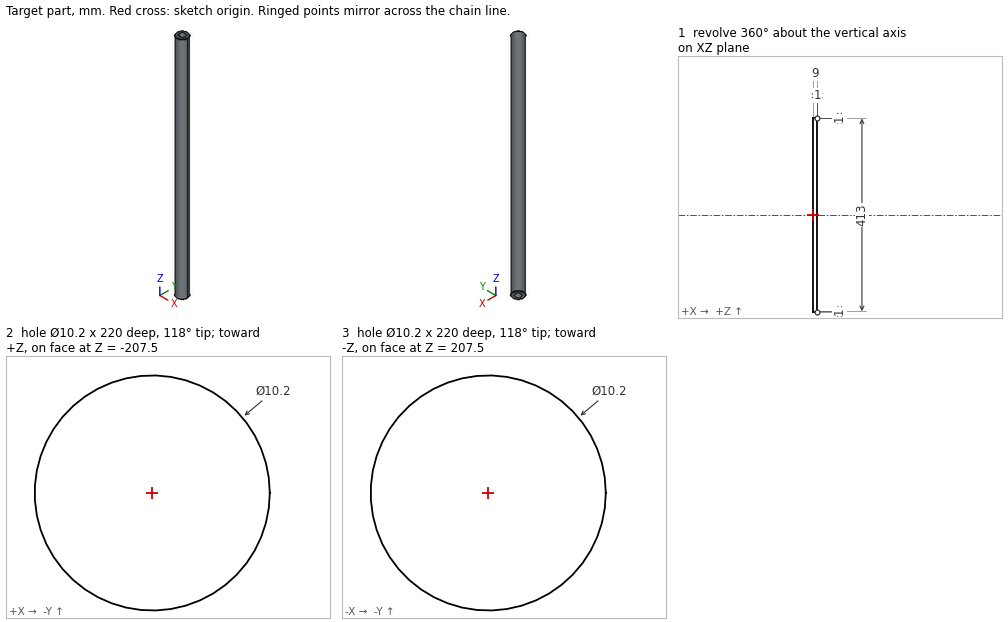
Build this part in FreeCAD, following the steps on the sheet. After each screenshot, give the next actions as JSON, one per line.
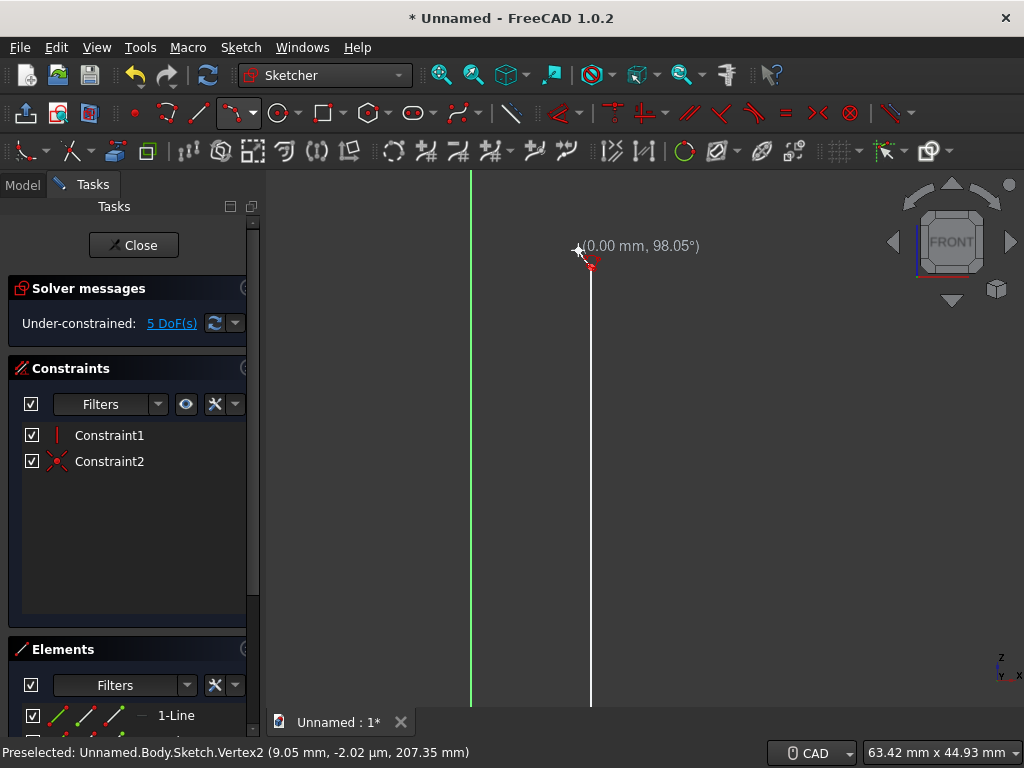
{"action": "scroll", "coordinate": [580, 255], "scroll_direction": "down", "scroll_amount": 13}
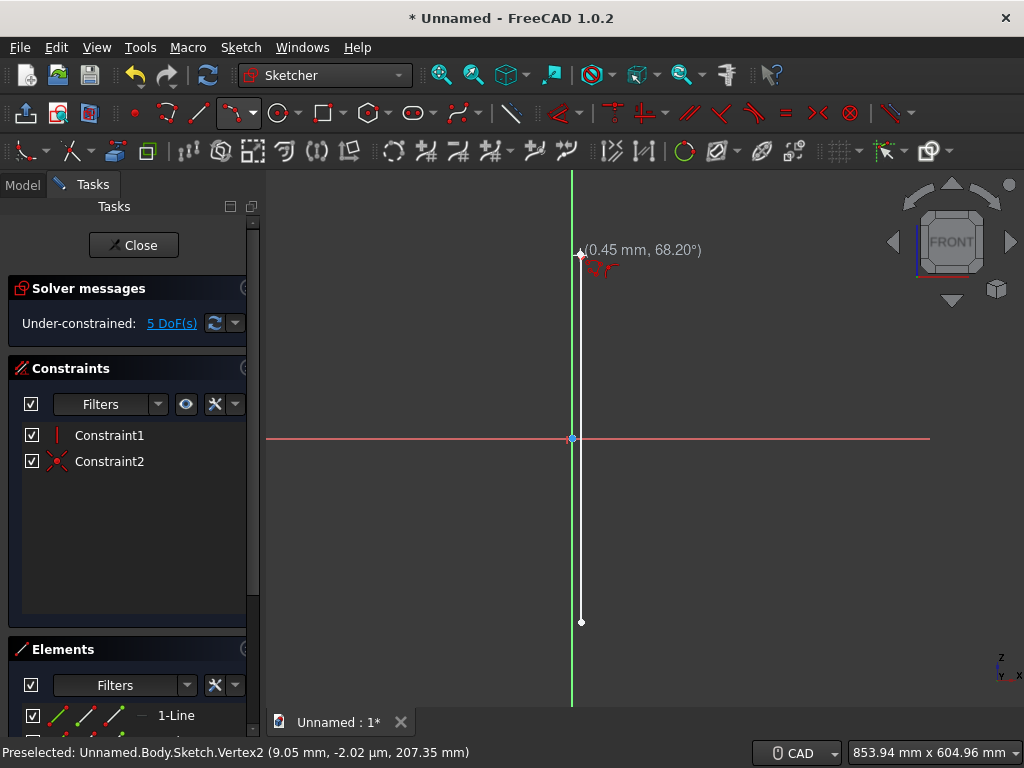
{"action": "scroll", "coordinate": [572, 255], "scroll_direction": "up", "scroll_amount": 4}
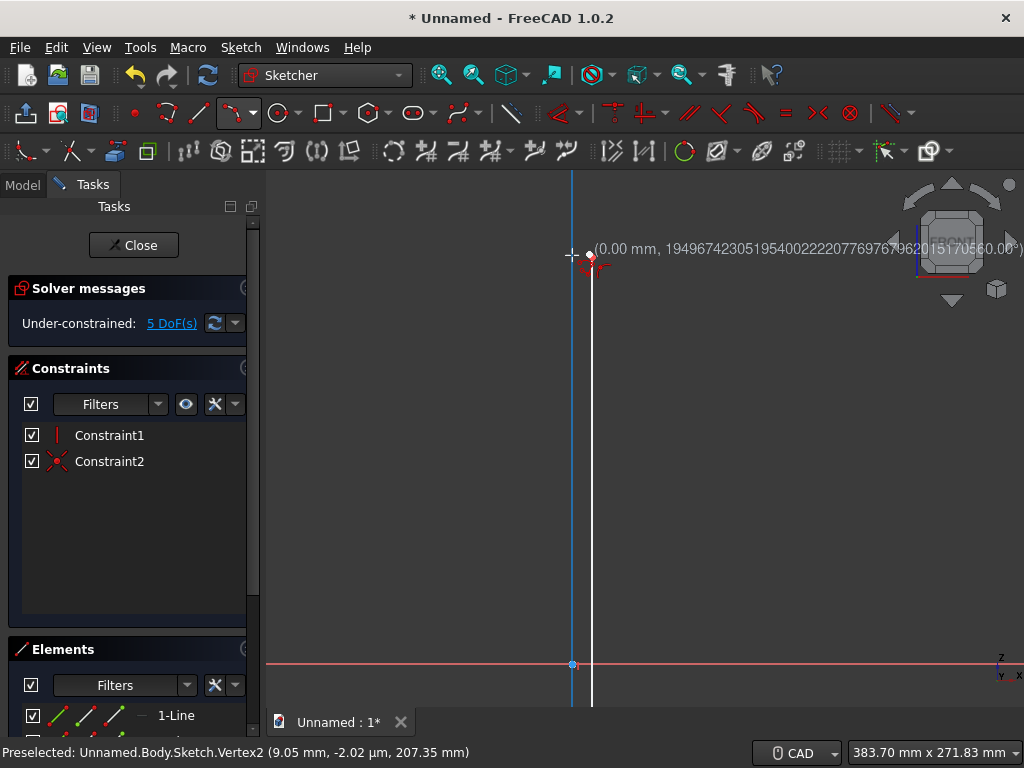
{"action": "left_click", "coordinate": [572, 254]}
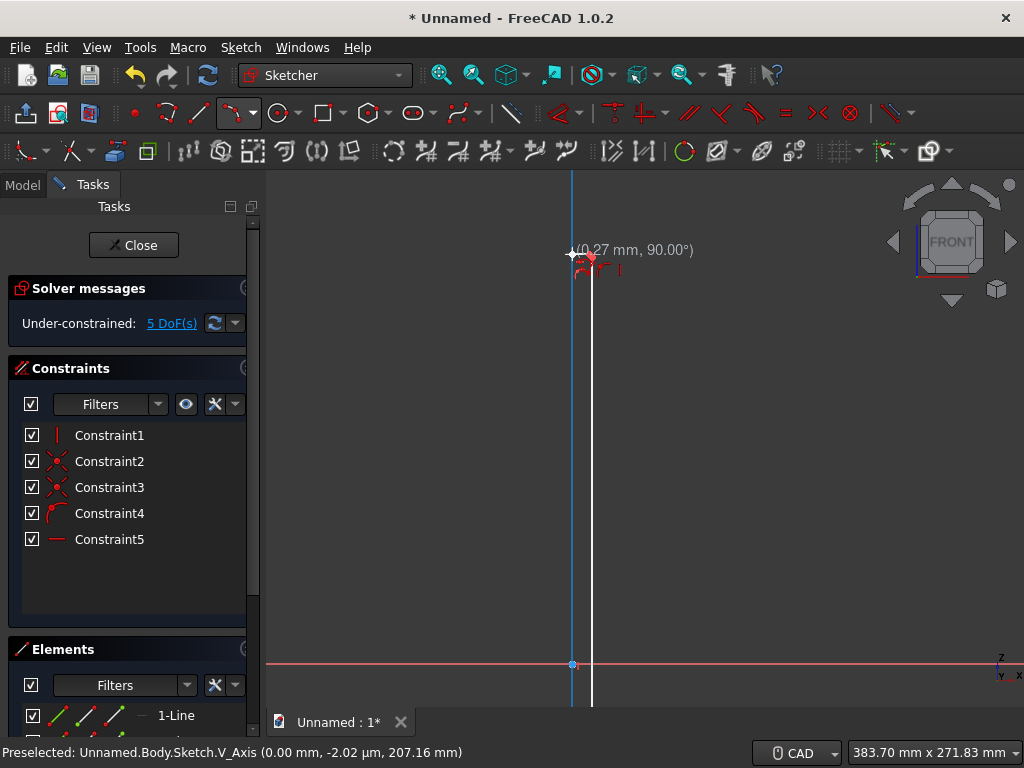
{"action": "scroll", "coordinate": [572, 254], "scroll_direction": "down", "scroll_amount": 4}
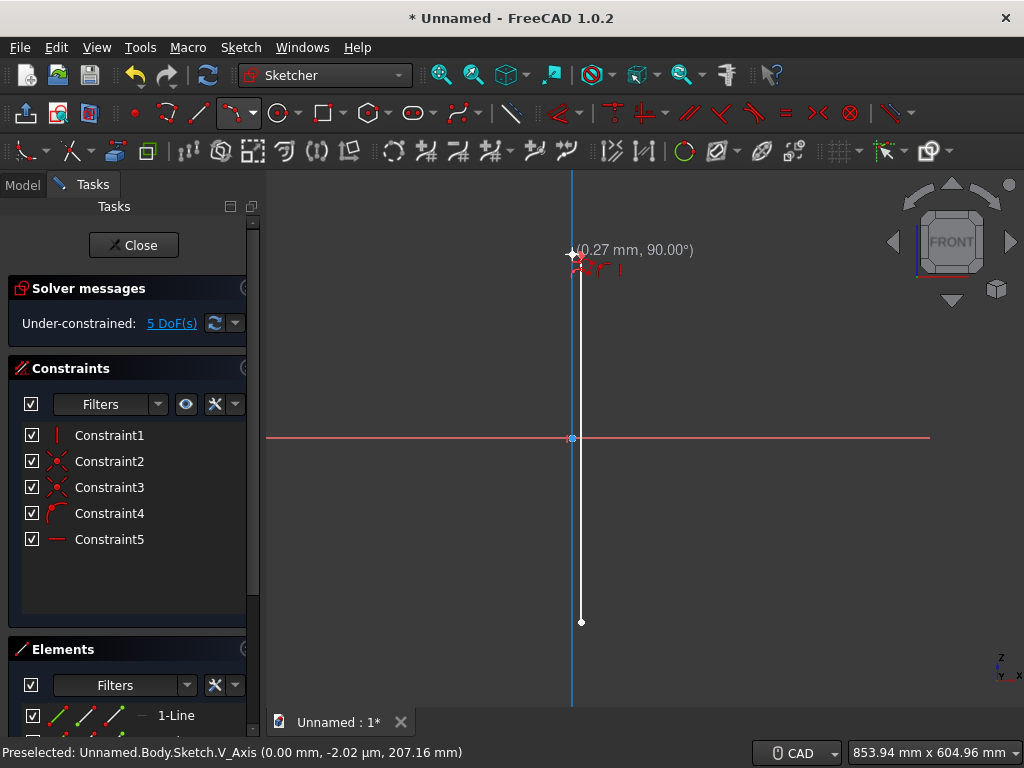
{"action": "scroll", "coordinate": [572, 623], "scroll_direction": "up", "scroll_amount": 3}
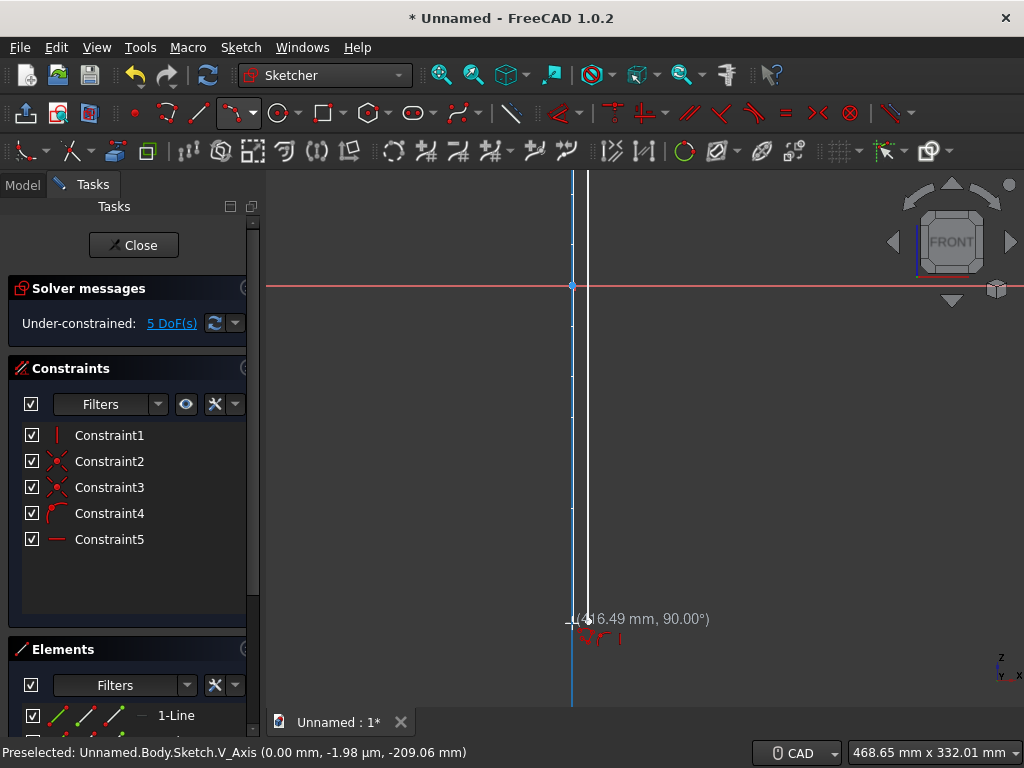
{"action": "left_click", "coordinate": [581, 622]}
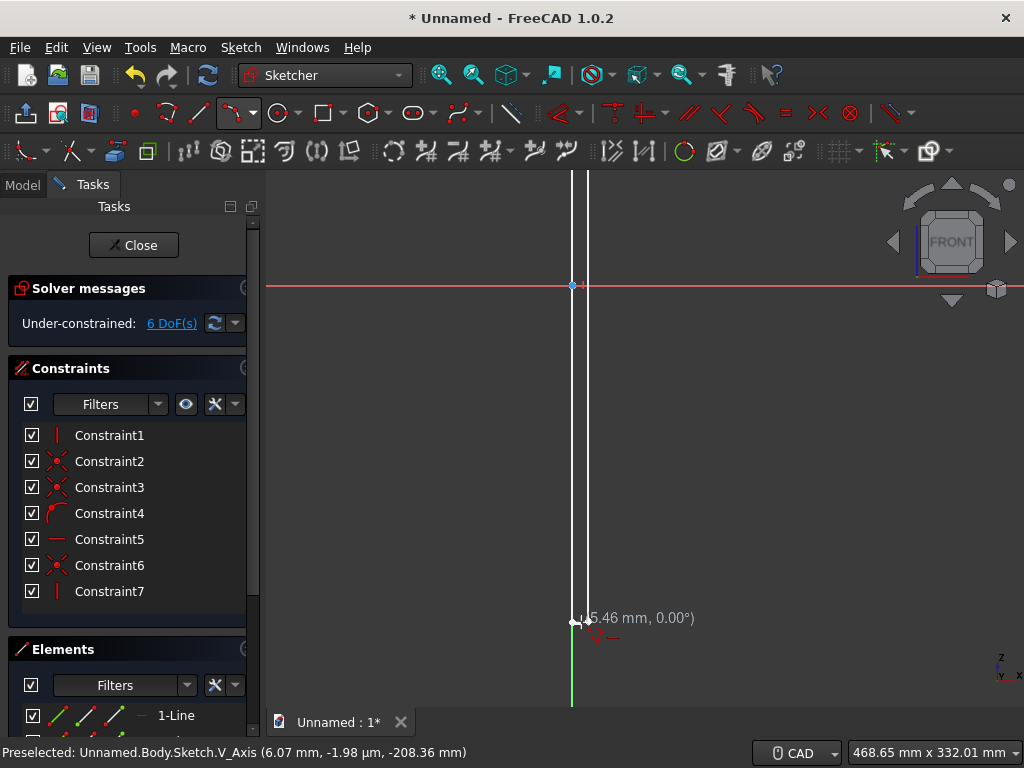
{"action": "scroll", "coordinate": [587, 622], "scroll_direction": "up", "scroll_amount": 10}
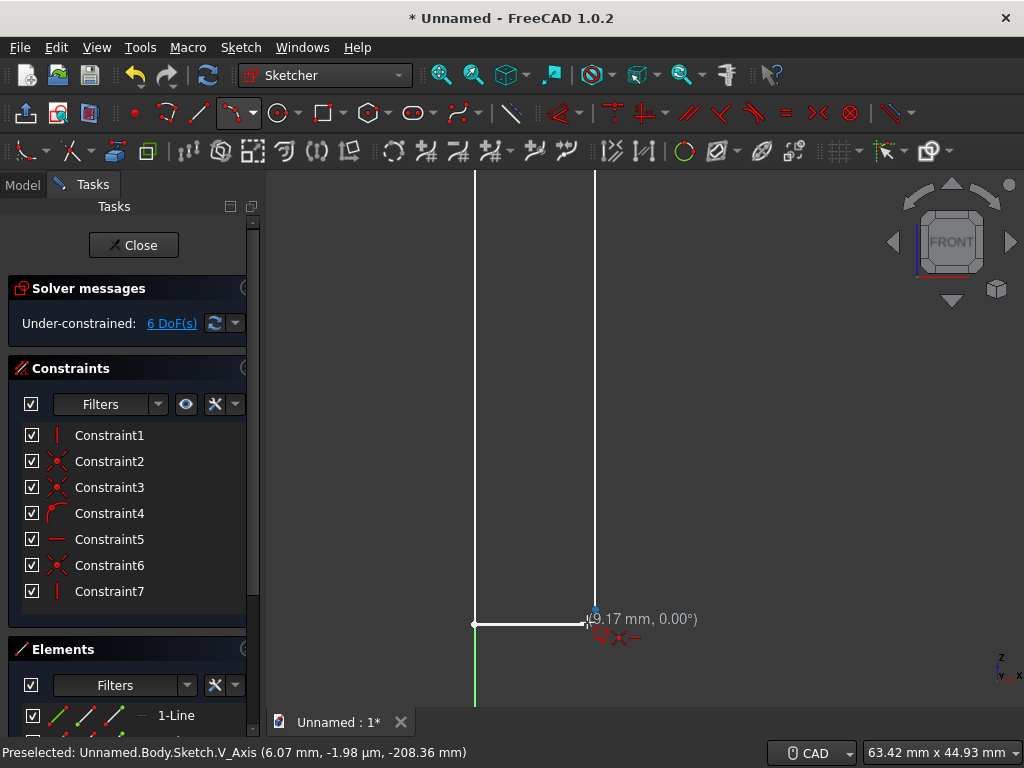
{"action": "left_click", "coordinate": [582, 617]}
{"action": "left_click", "coordinate": [595, 609]}
{"action": "key", "text": "Escape"}
{"action": "key", "text": "Escape"}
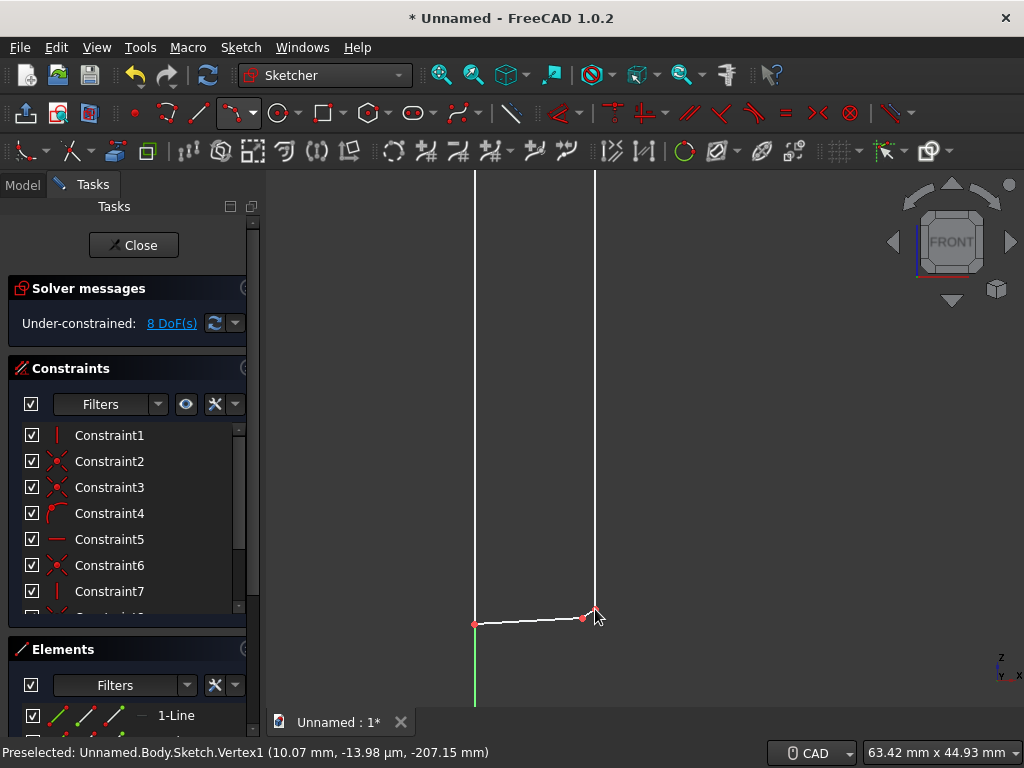
{"action": "left_click", "coordinate": [507, 622]}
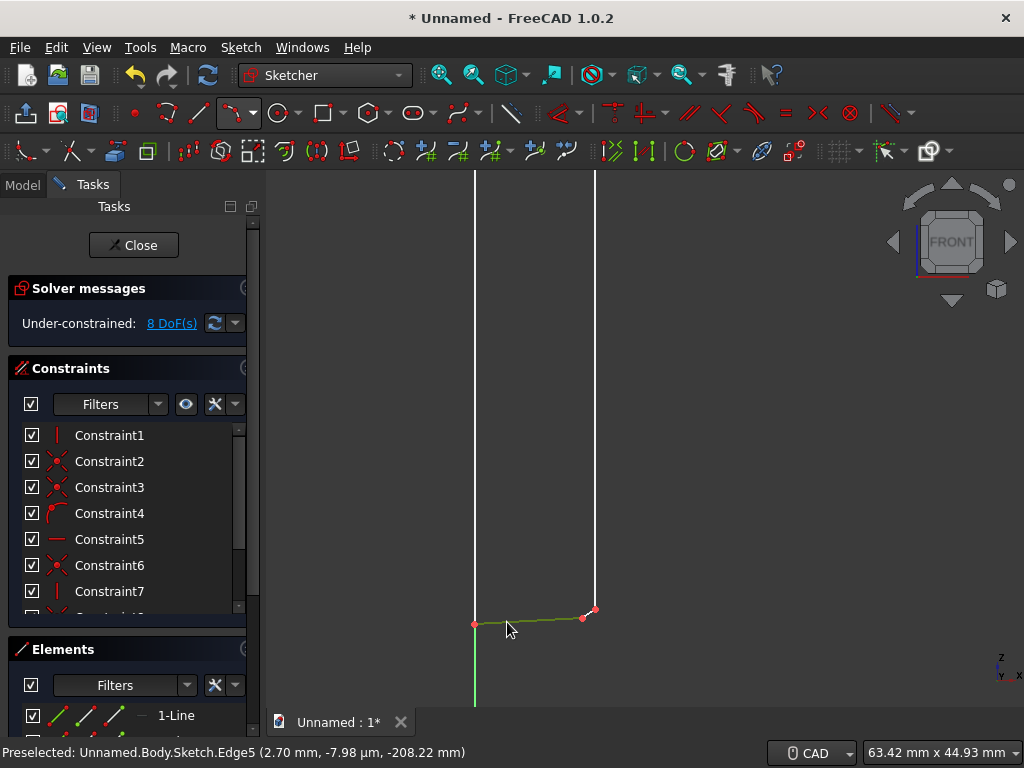
{"action": "key", "text": "h"}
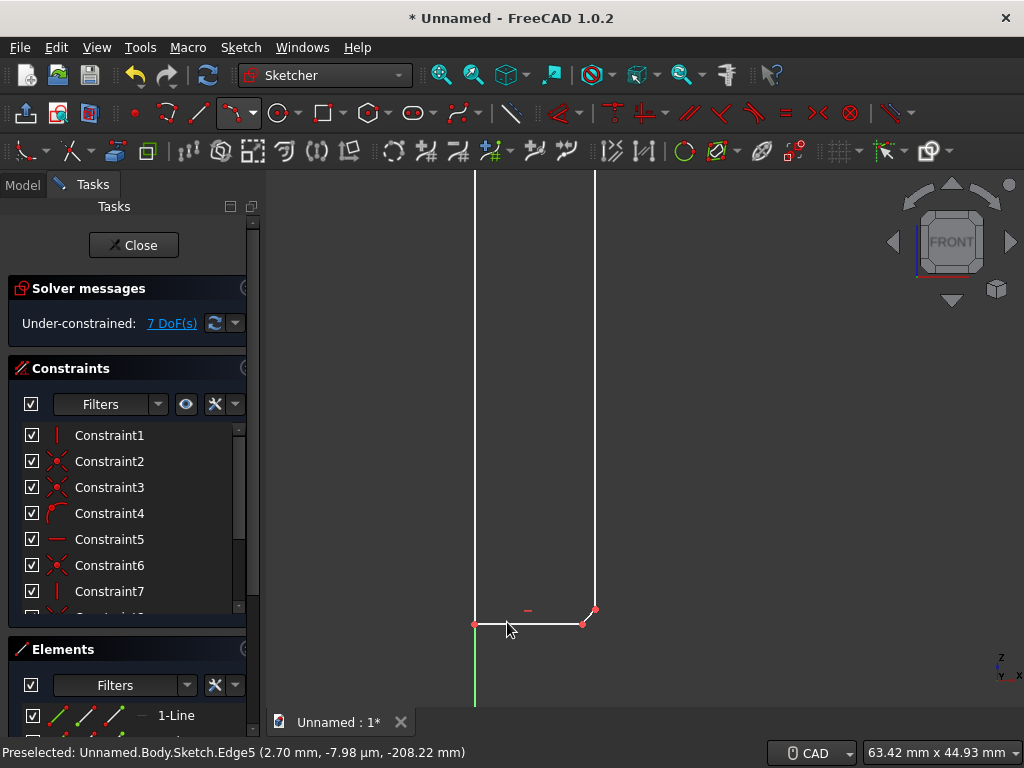
{"action": "scroll", "coordinate": [580, 623], "scroll_direction": "down", "scroll_amount": 13}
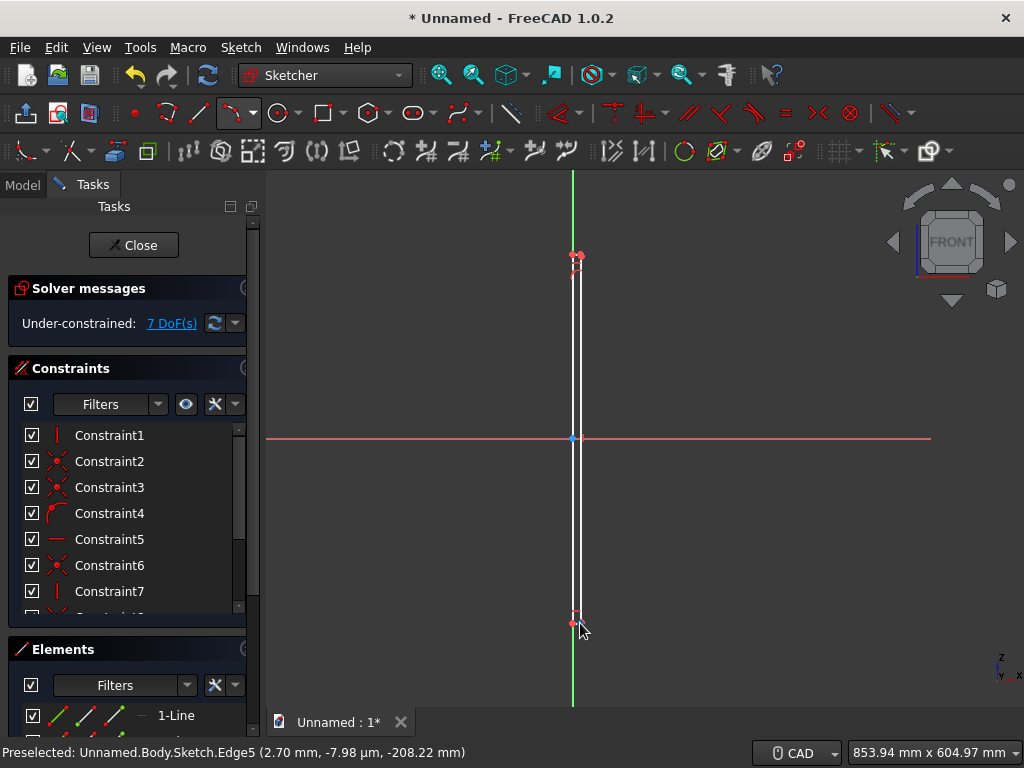
{"action": "scroll", "coordinate": [581, 255], "scroll_direction": "up", "scroll_amount": 11}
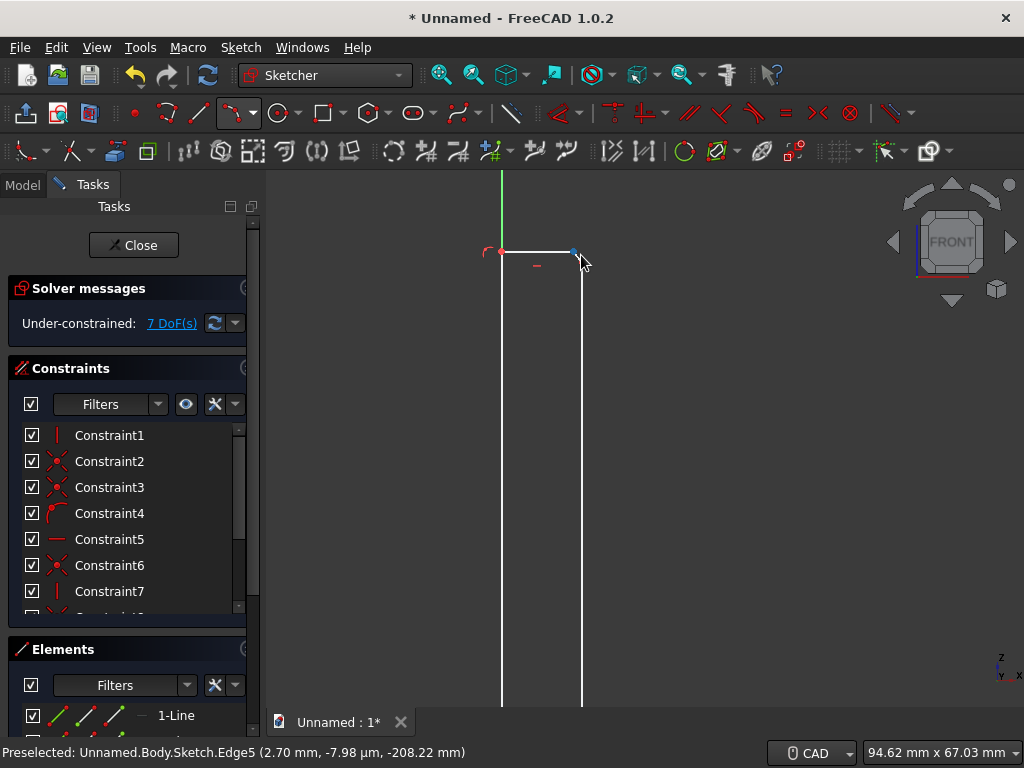
{"action": "left_click", "coordinate": [573, 252]}